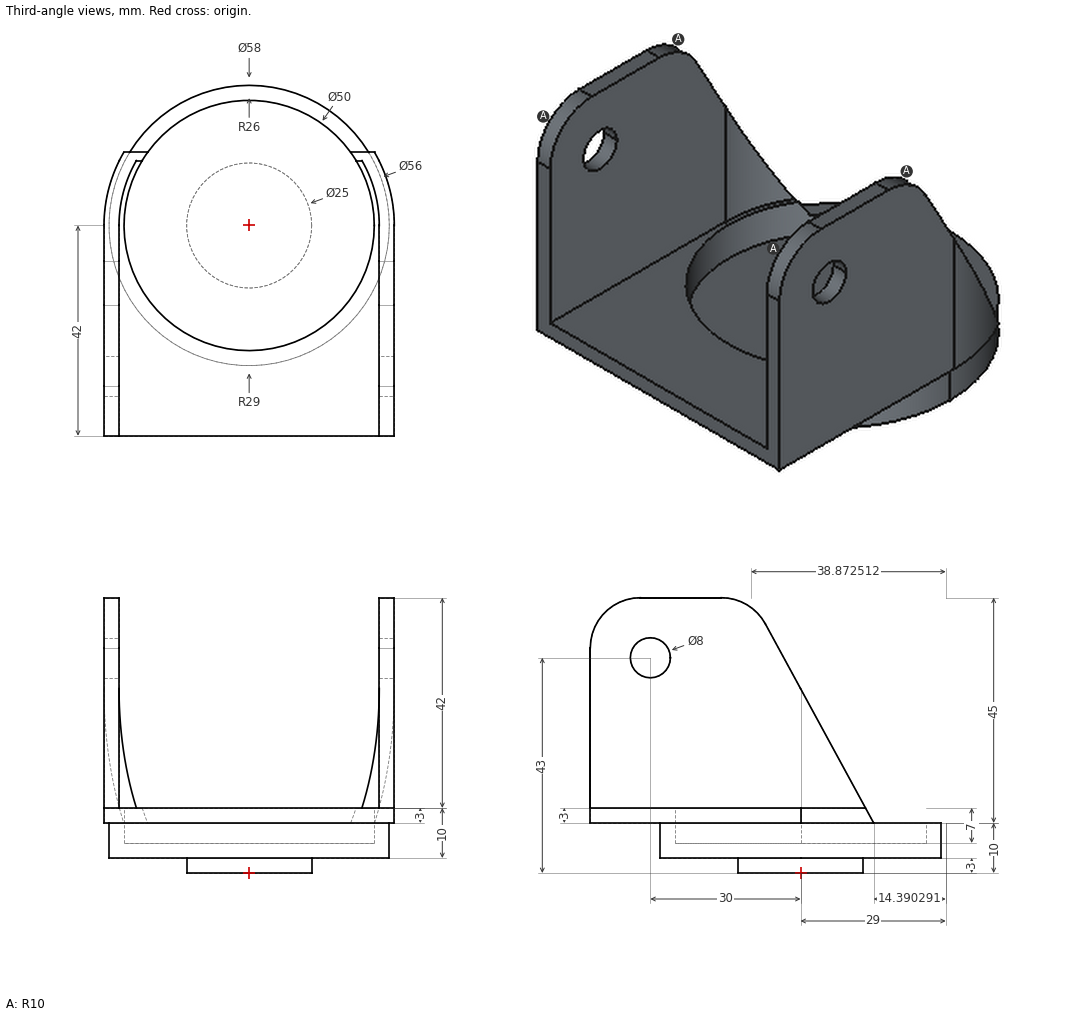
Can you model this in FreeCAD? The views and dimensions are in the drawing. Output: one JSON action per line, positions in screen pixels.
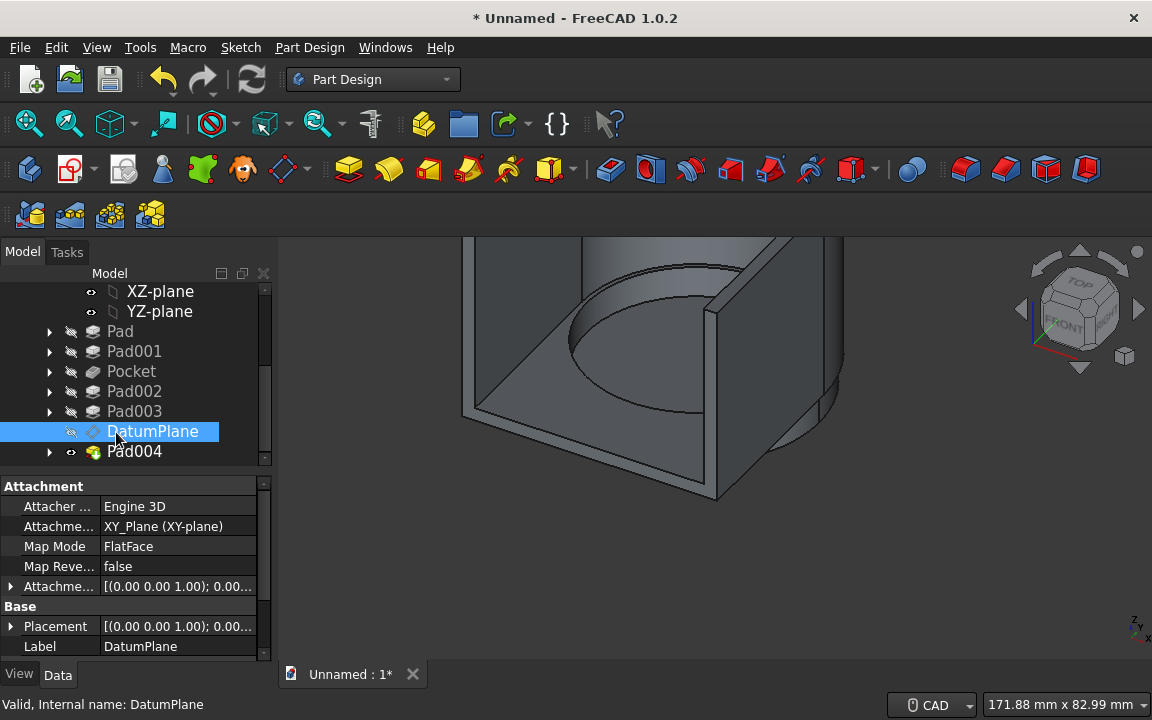
{"action": "left_click", "coordinate": [30, 124]}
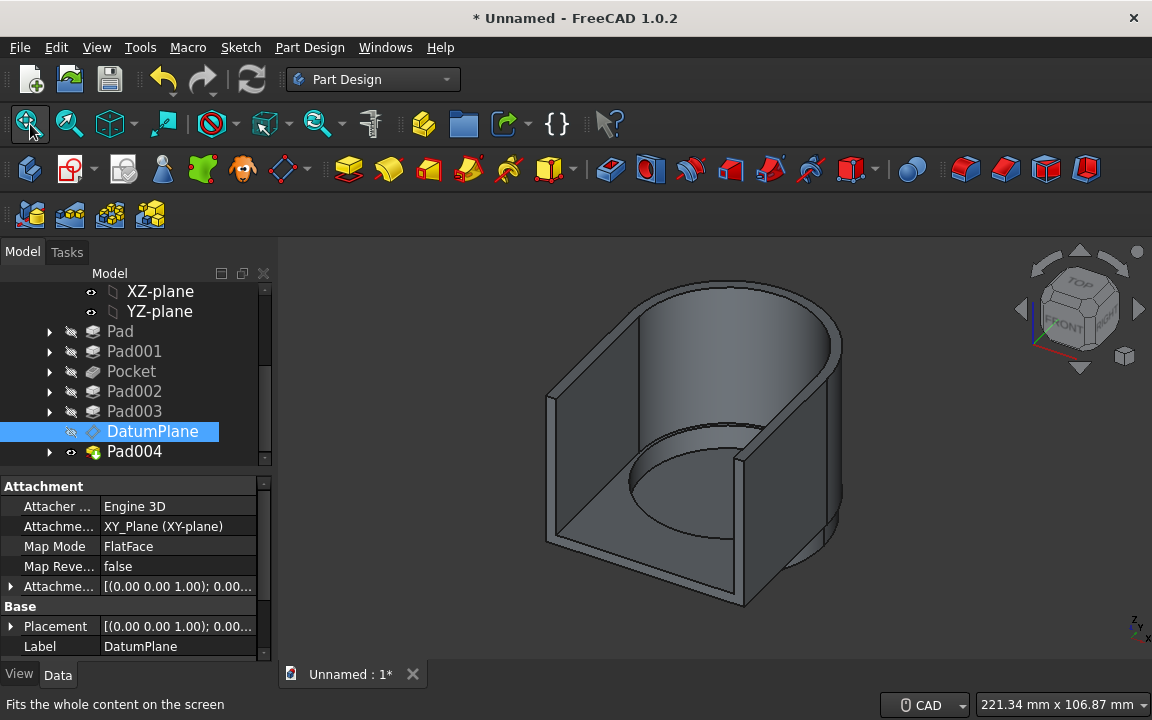
{"action": "left_click", "coordinate": [786, 492]}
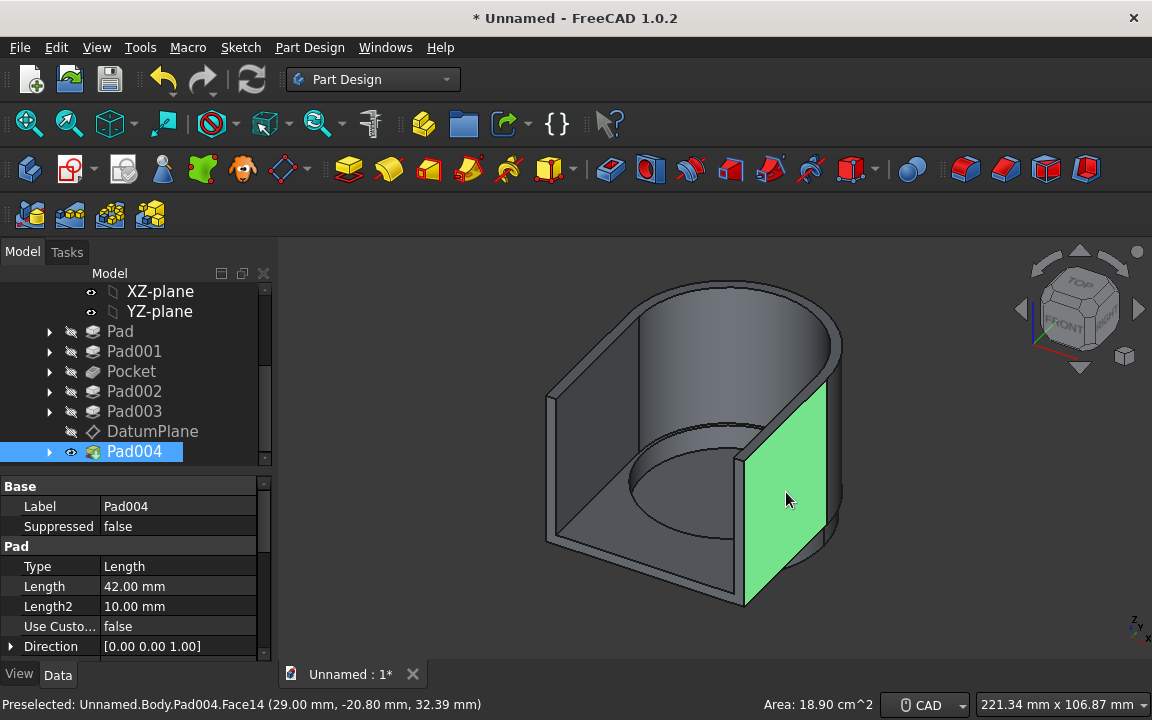
{"action": "left_click", "coordinate": [70, 170]}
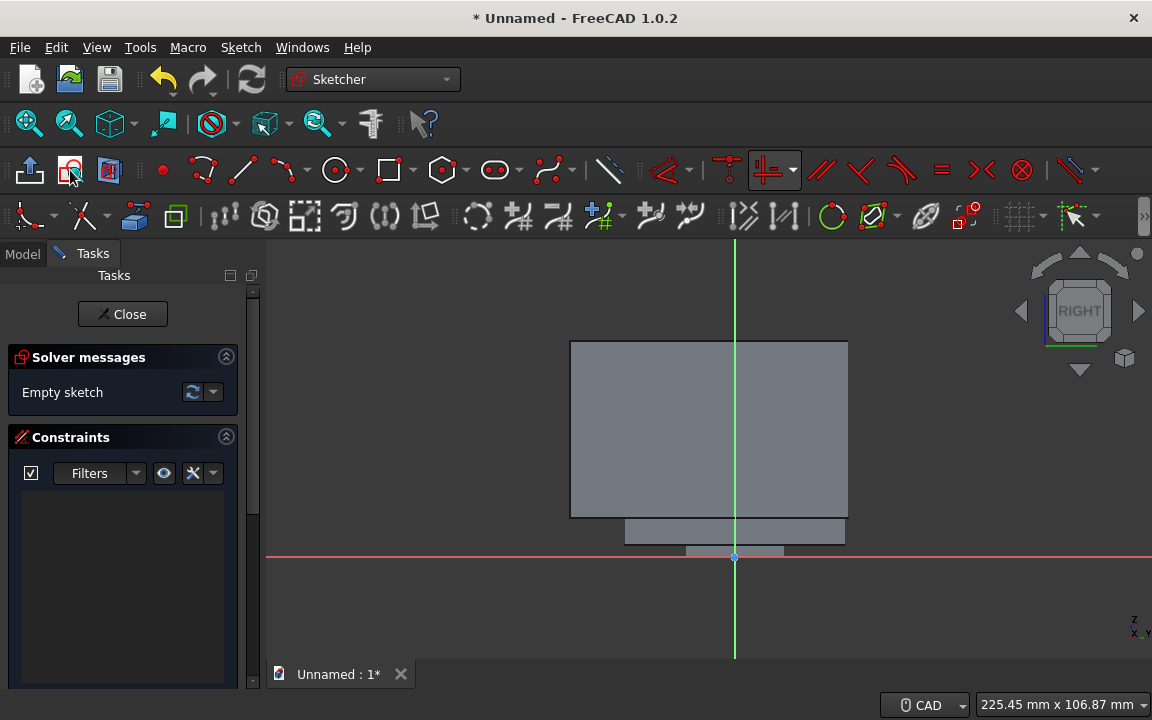
{"action": "left_click", "coordinate": [204, 170]}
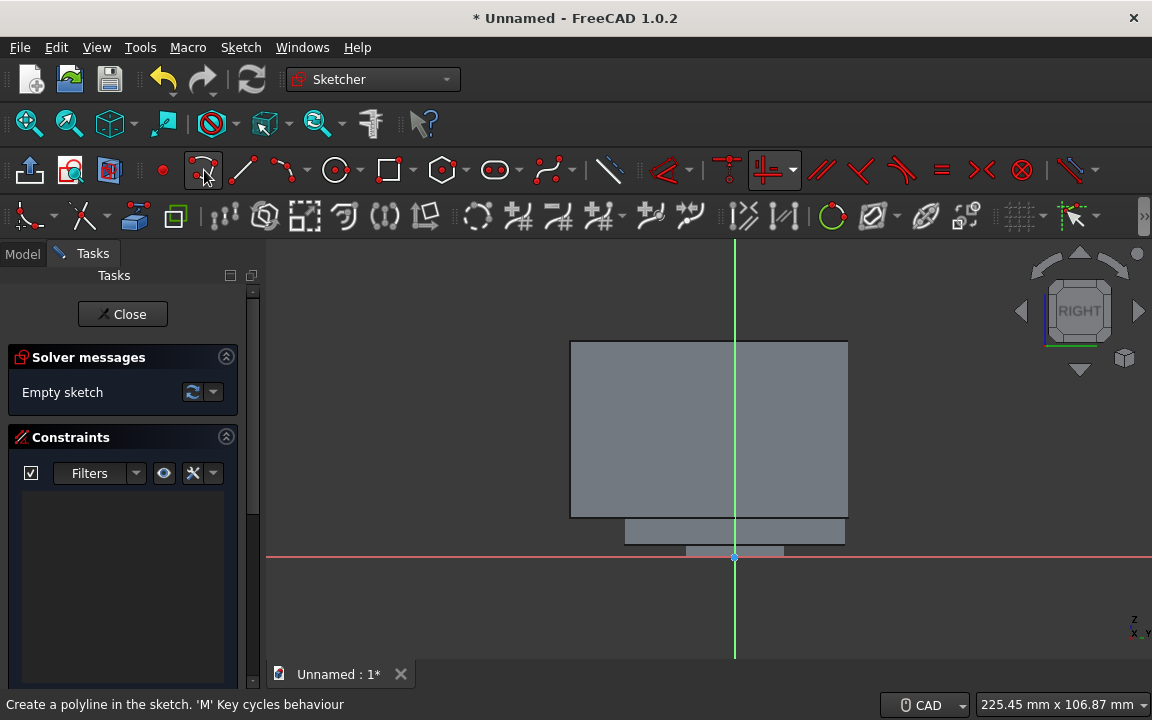
{"action": "left_click", "coordinate": [792, 518]}
{"action": "left_click", "coordinate": [849, 518]}
{"action": "left_click", "coordinate": [849, 341]}
{"action": "left_click", "coordinate": [696, 341]}
{"action": "left_click", "coordinate": [792, 519]}
{"action": "key", "text": "Escape"}
{"action": "key", "text": "Escape"}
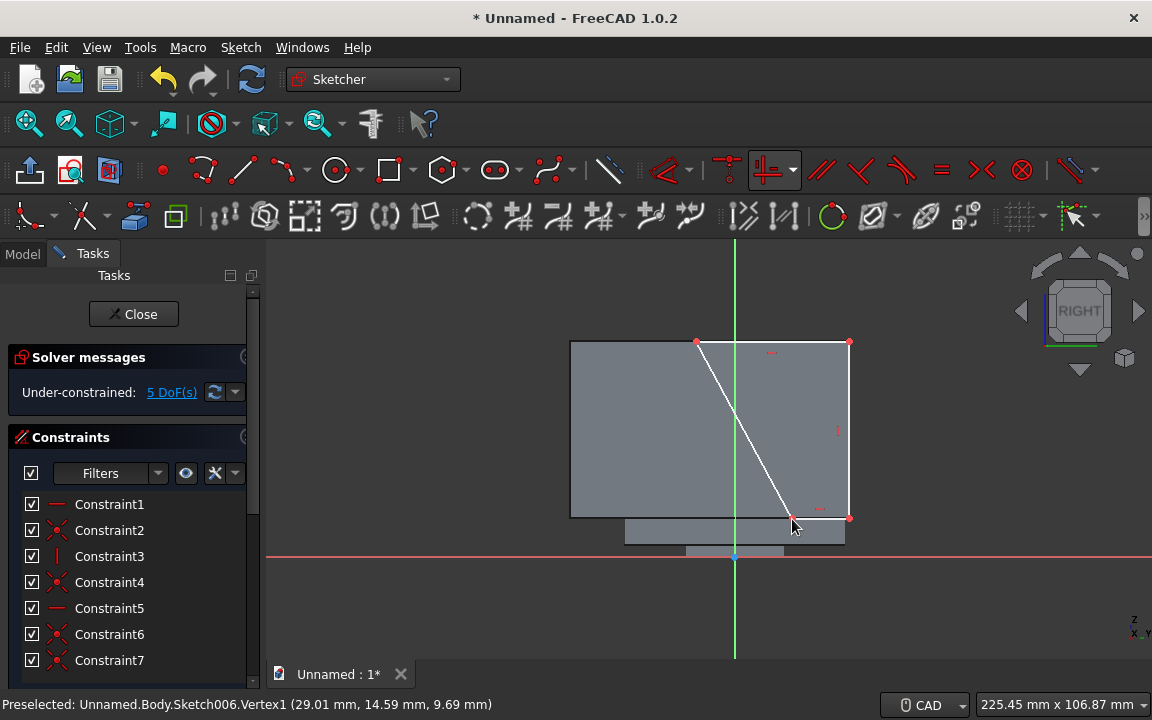
{"action": "left_click", "coordinate": [664, 170]}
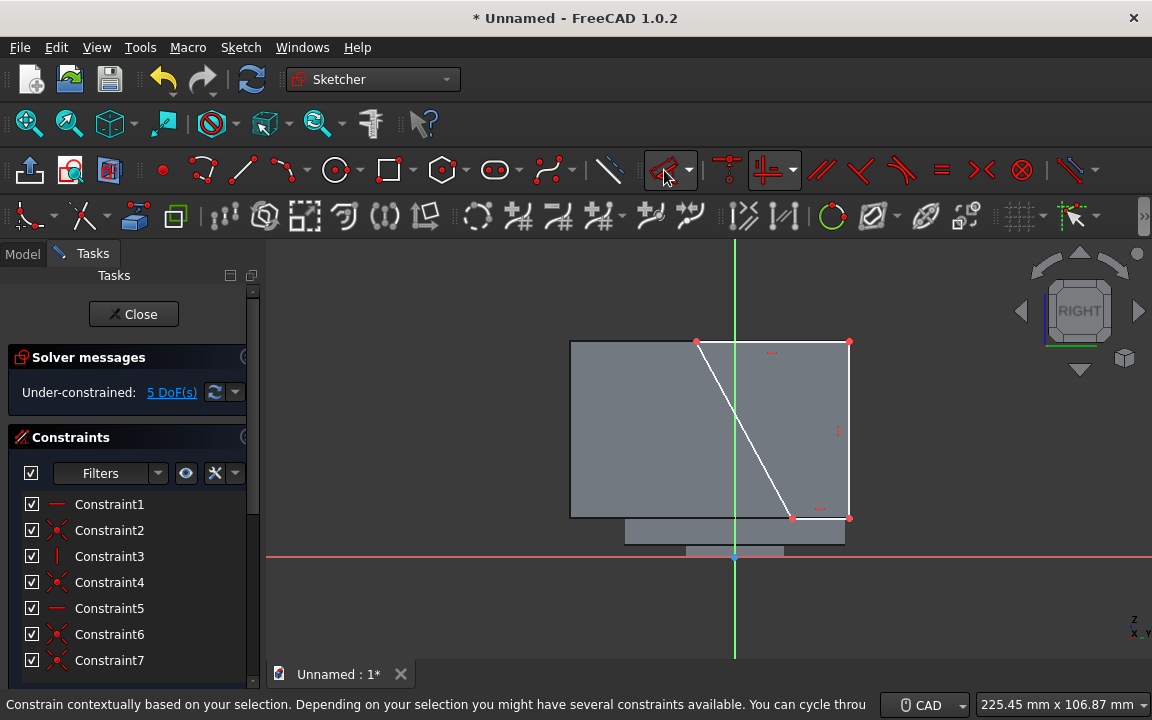
{"action": "left_click", "coordinate": [849, 466]}
{"action": "left_click", "coordinate": [883, 430]}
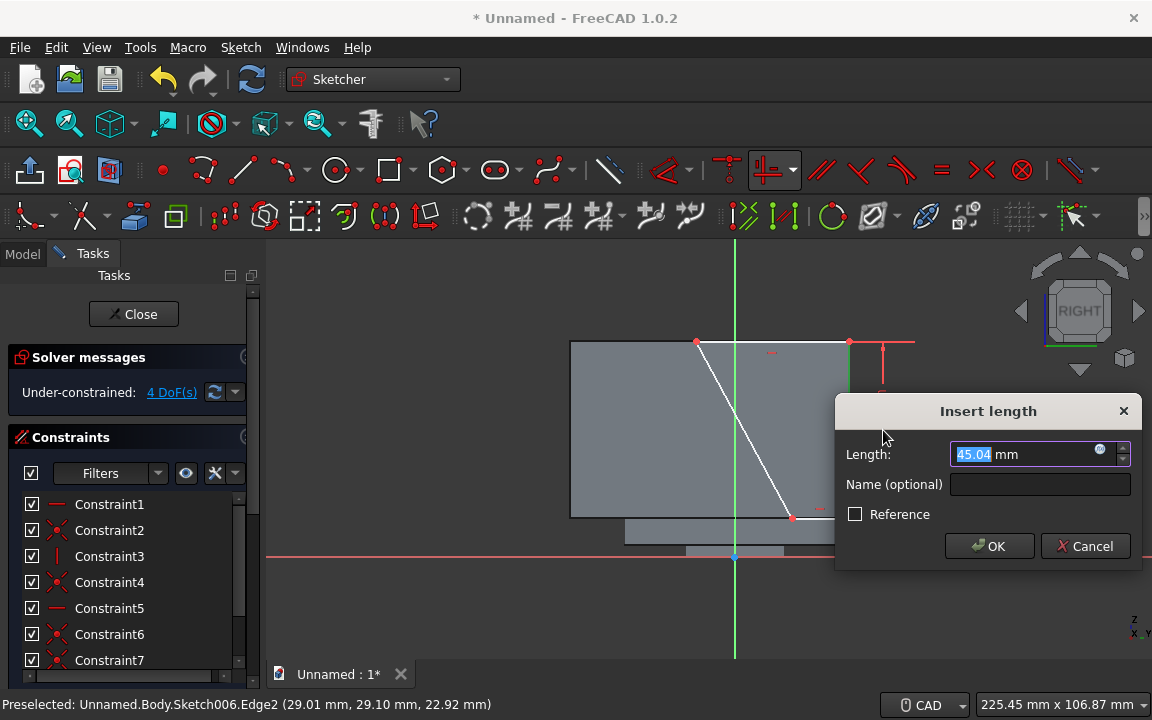
{"action": "type", "text": "45"}
{"action": "key", "text": "Return"}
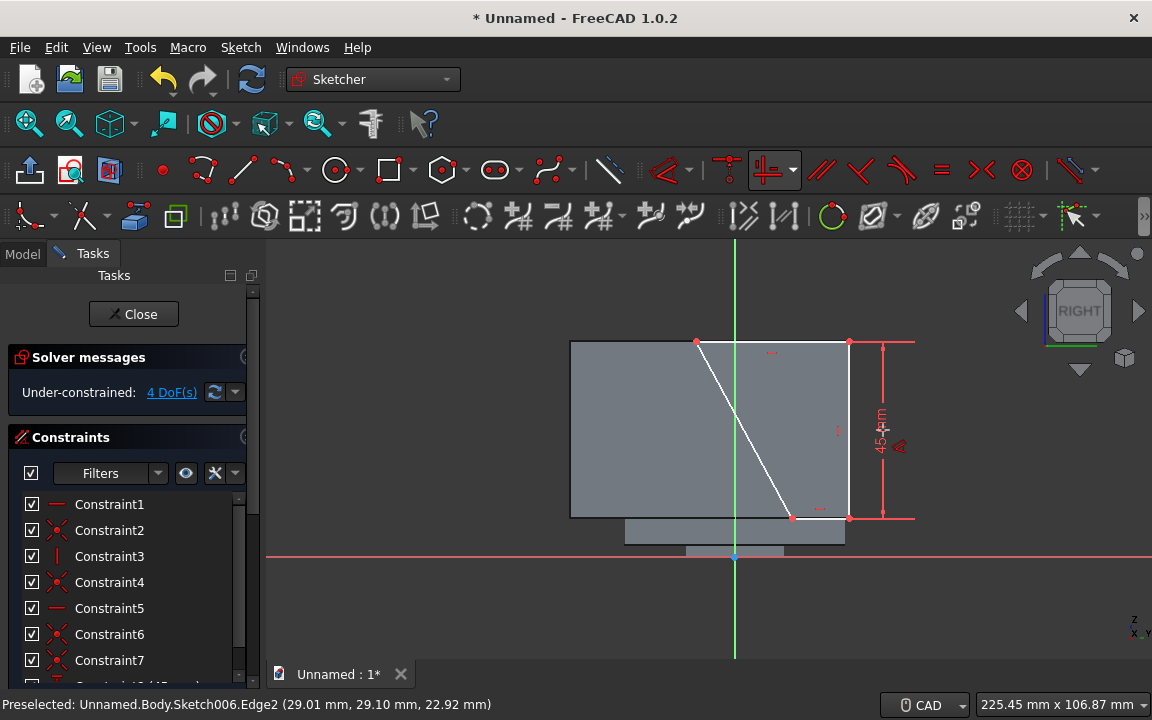
{"action": "left_click", "coordinate": [792, 519]}
{"action": "left_click", "coordinate": [701, 538]}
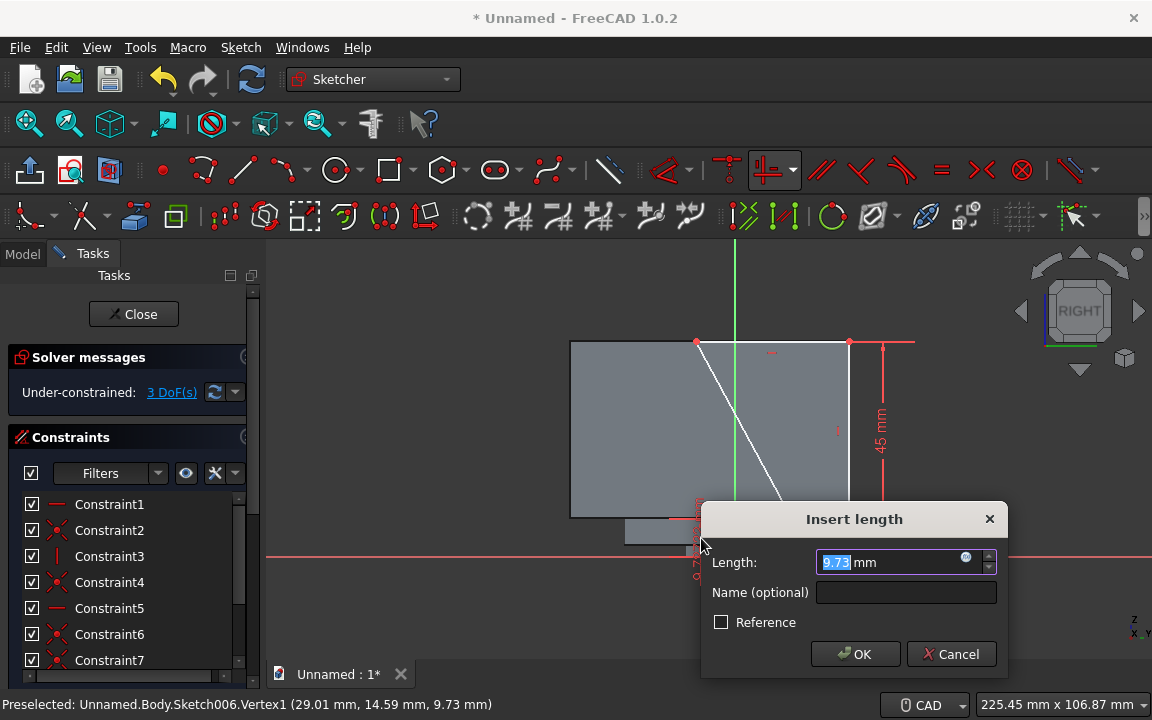
{"action": "type", "text": "10"}
{"action": "key", "text": "Return"}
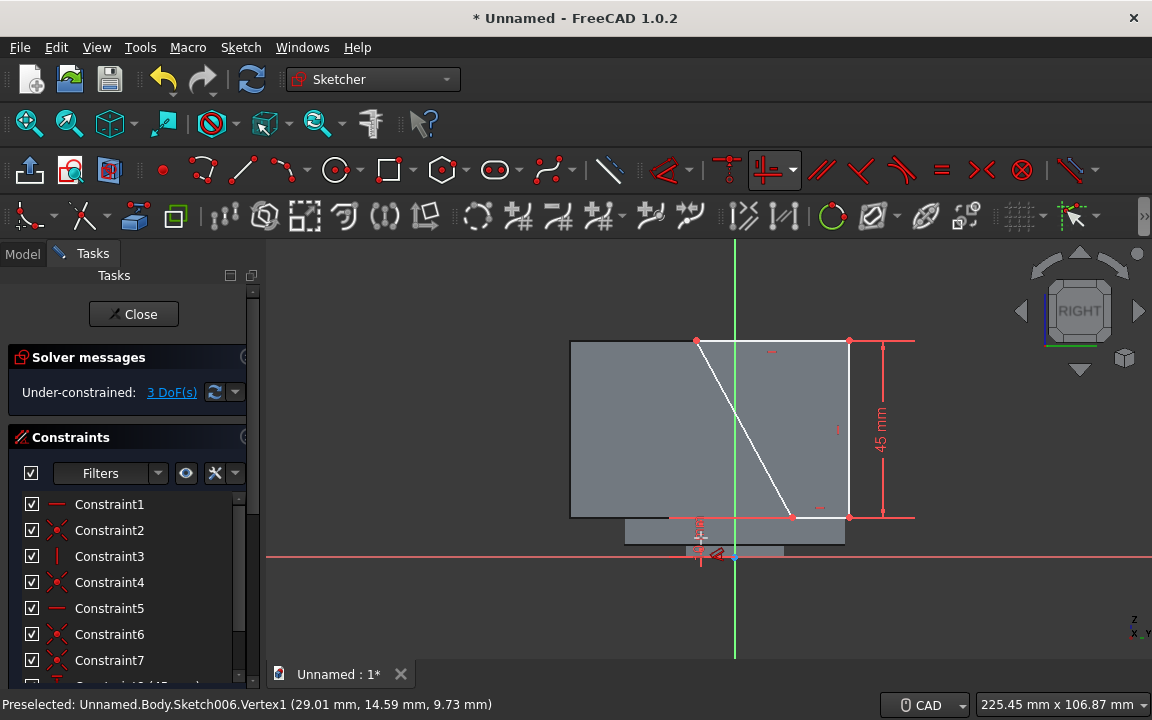
{"action": "left_click", "coordinate": [849, 518]}
{"action": "left_click", "coordinate": [792, 591]}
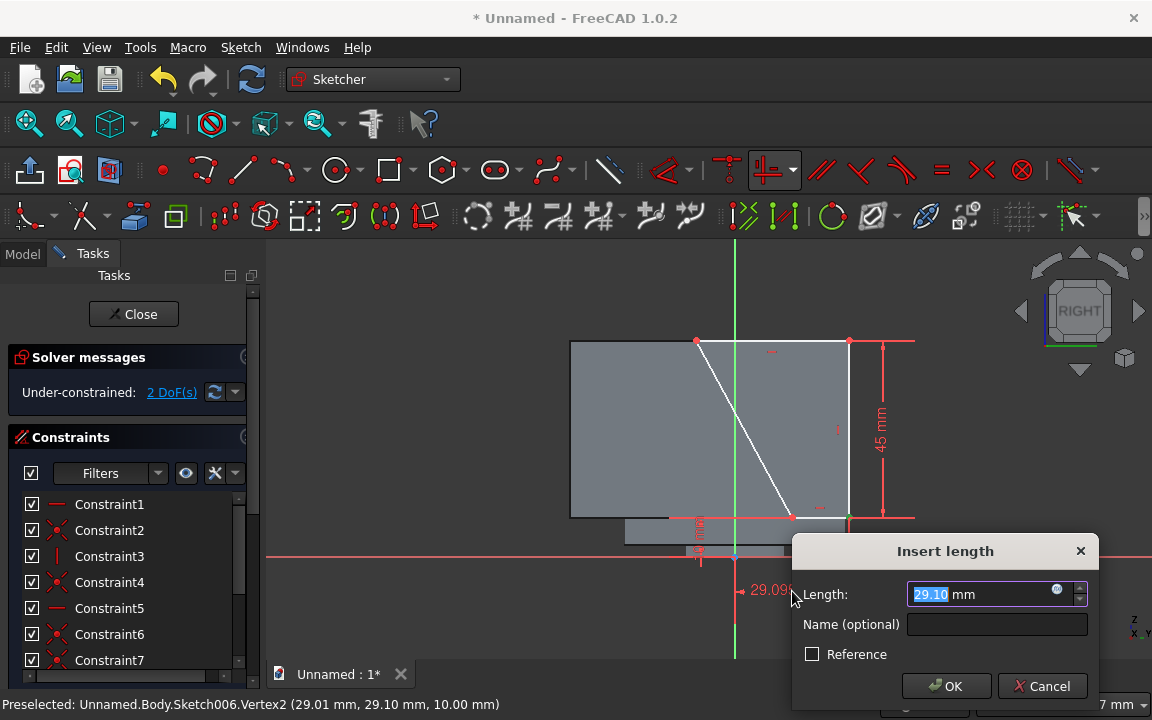
{"action": "type", "text": "29"}
{"action": "key", "text": "Return"}